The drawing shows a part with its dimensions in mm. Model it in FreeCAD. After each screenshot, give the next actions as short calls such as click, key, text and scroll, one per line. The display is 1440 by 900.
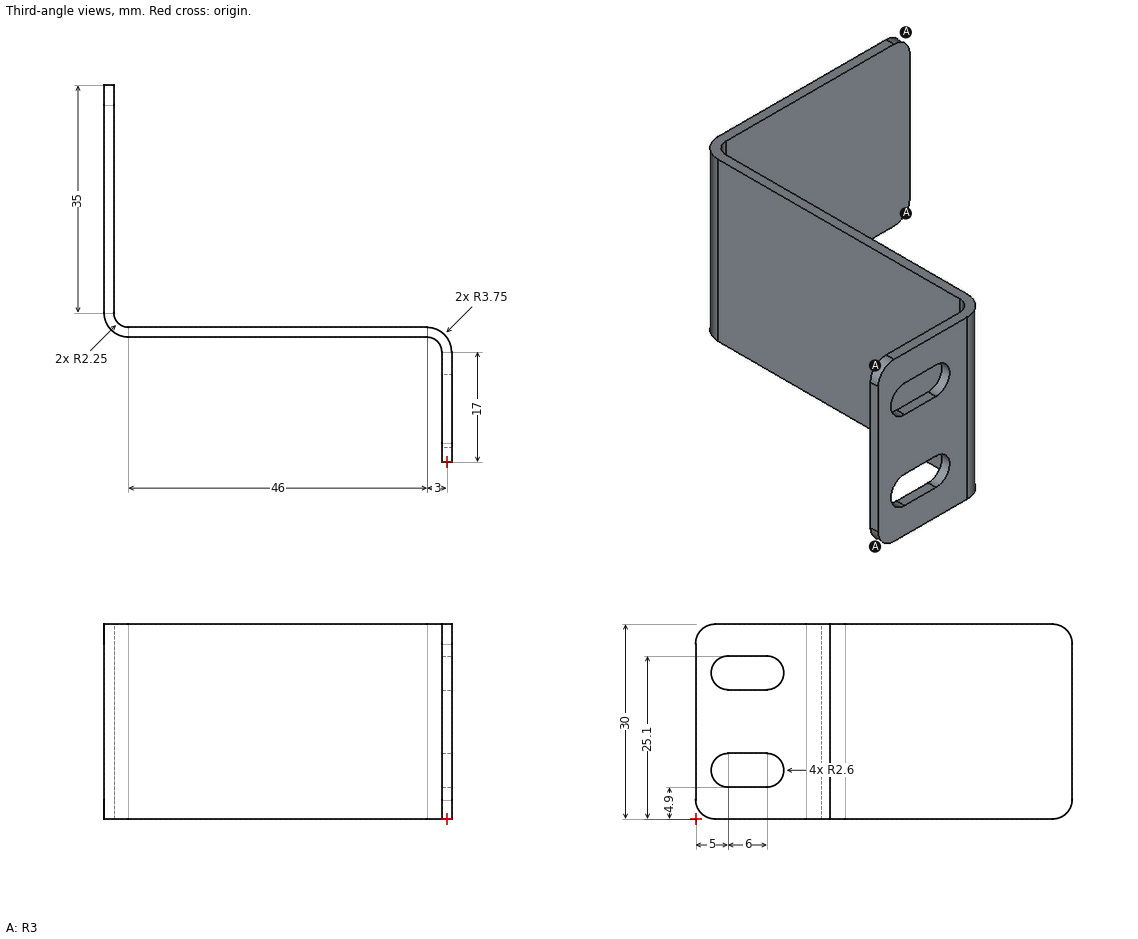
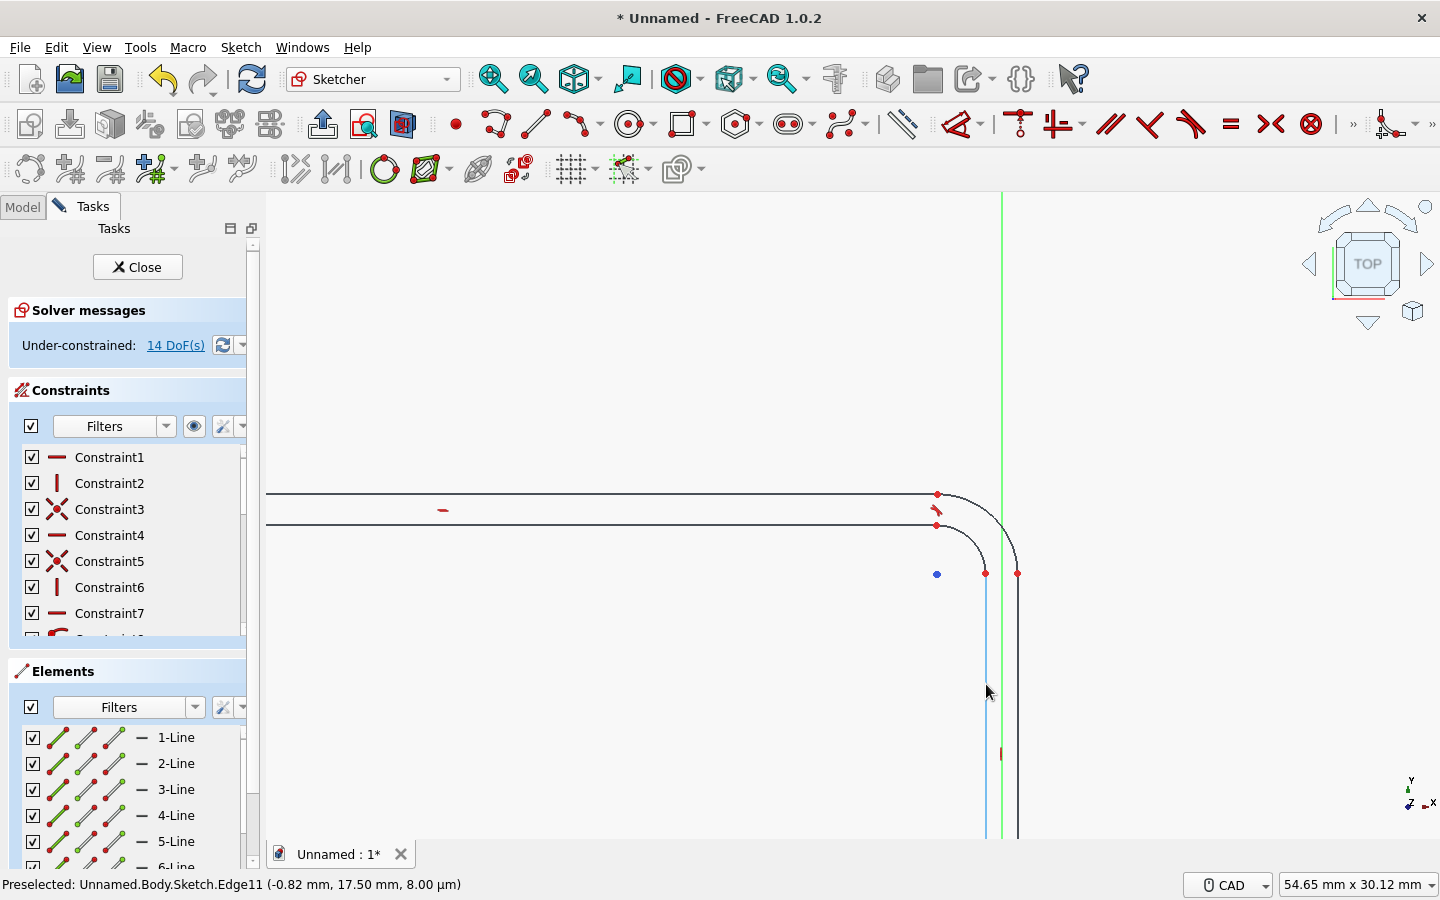
click(986, 683)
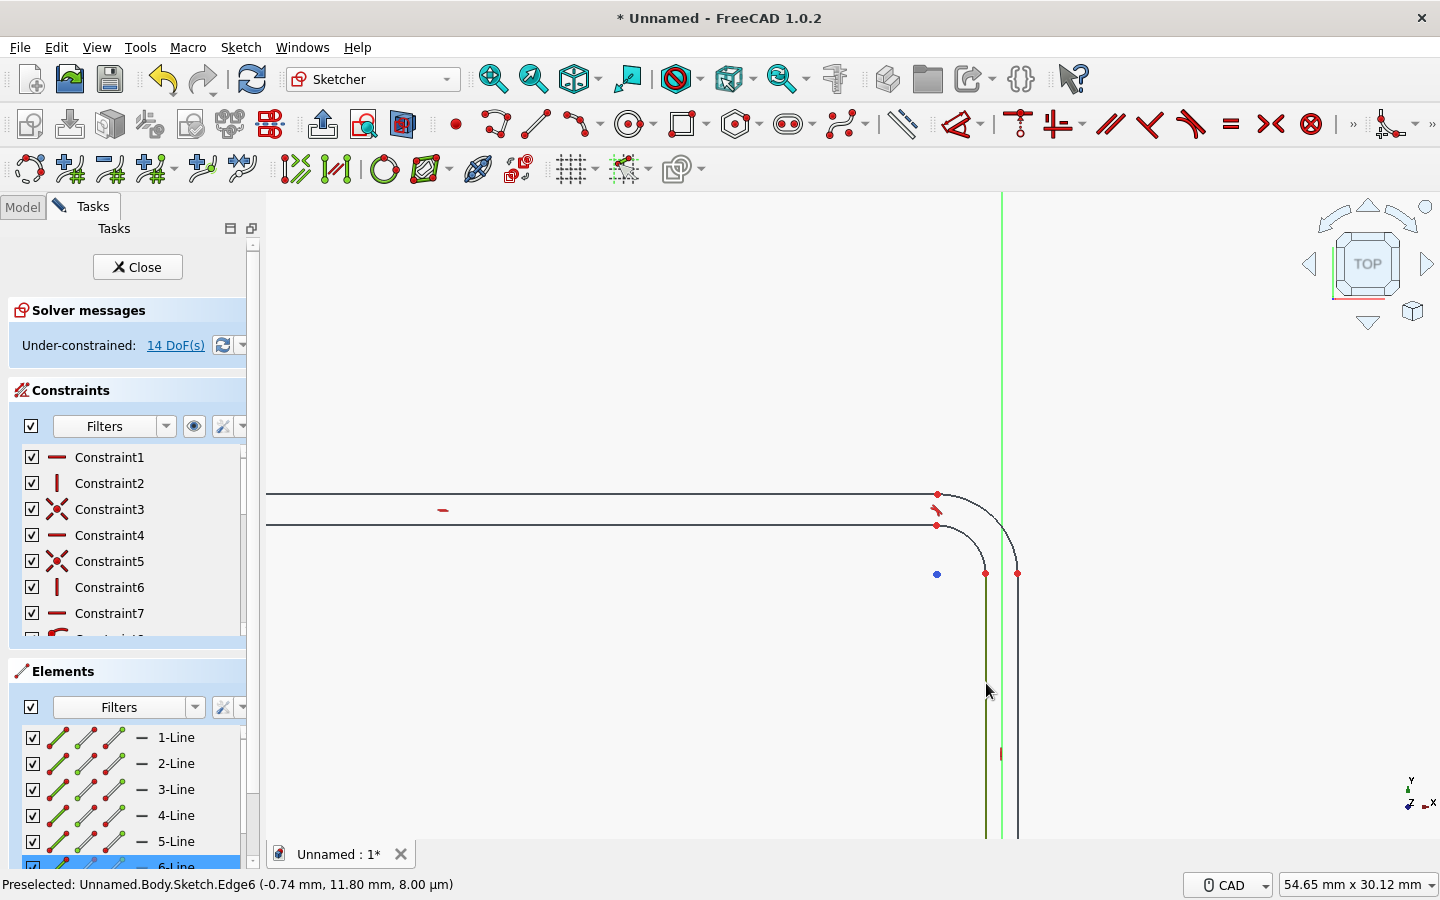
click(980, 552)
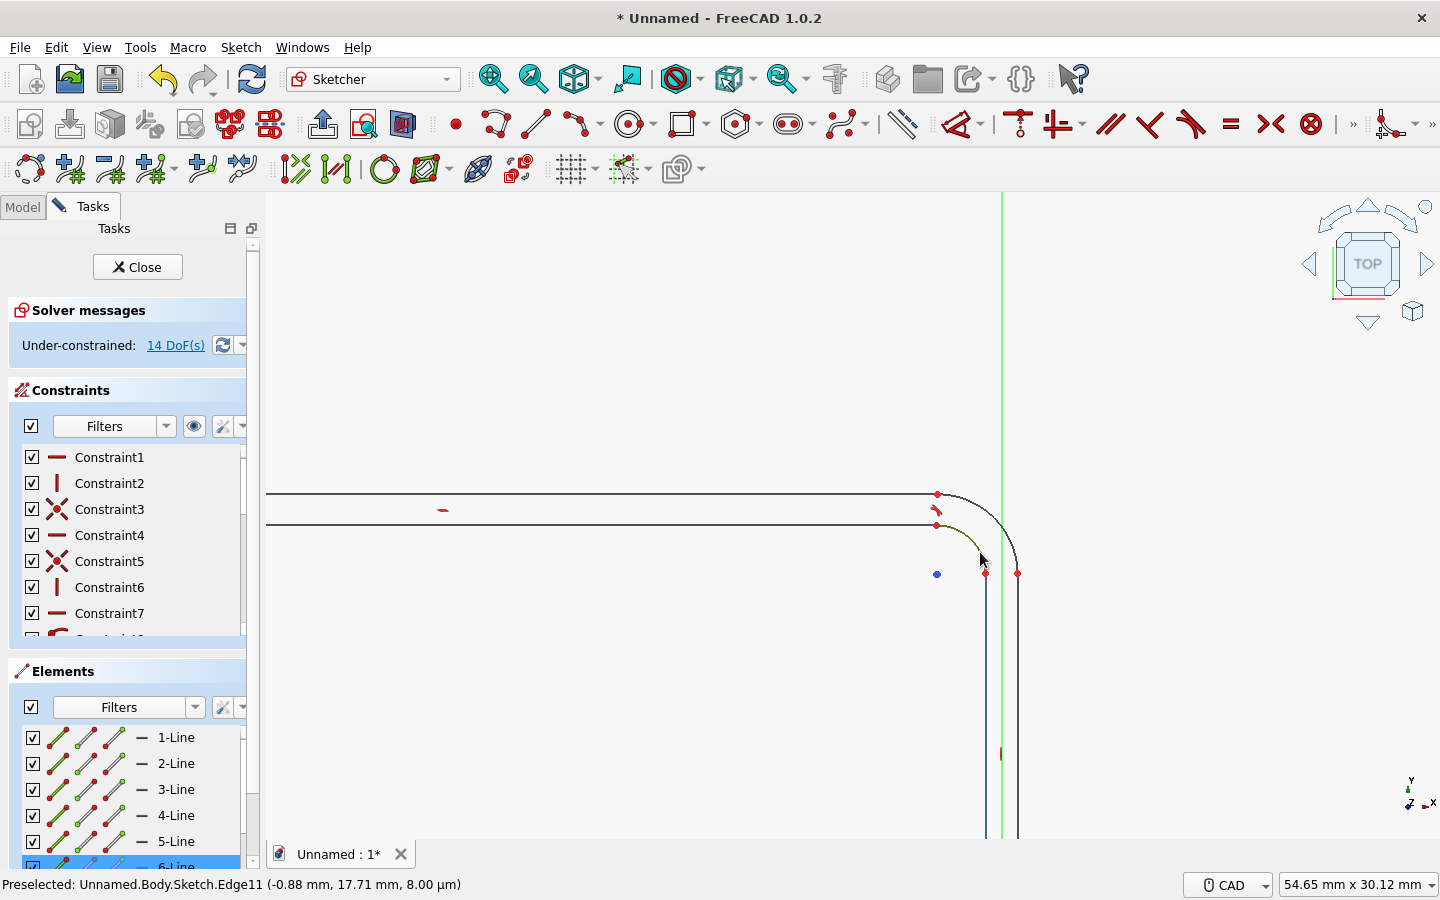
key(t)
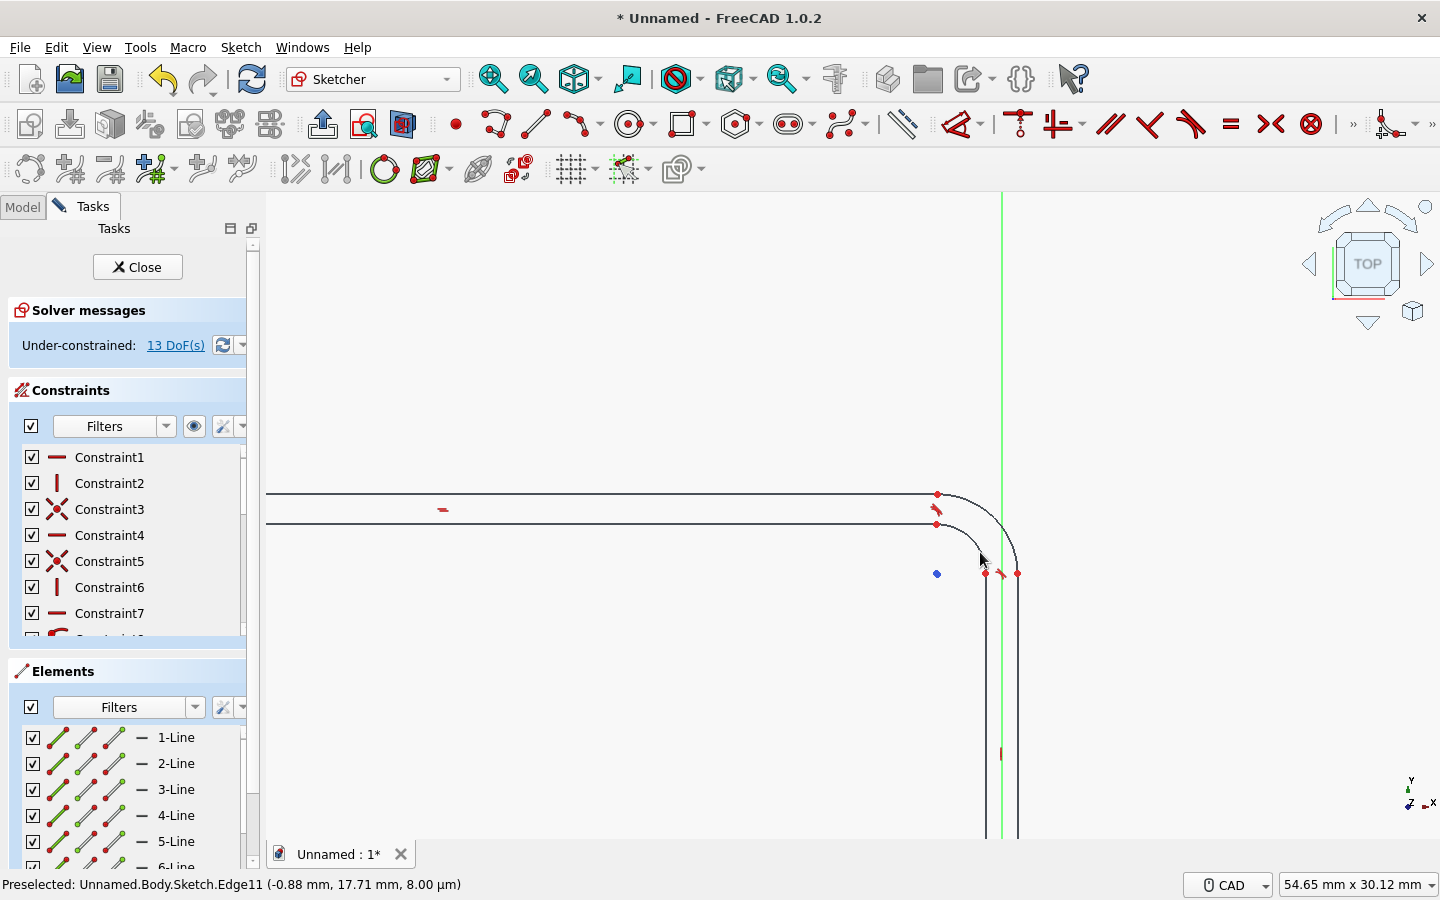
click(1018, 681)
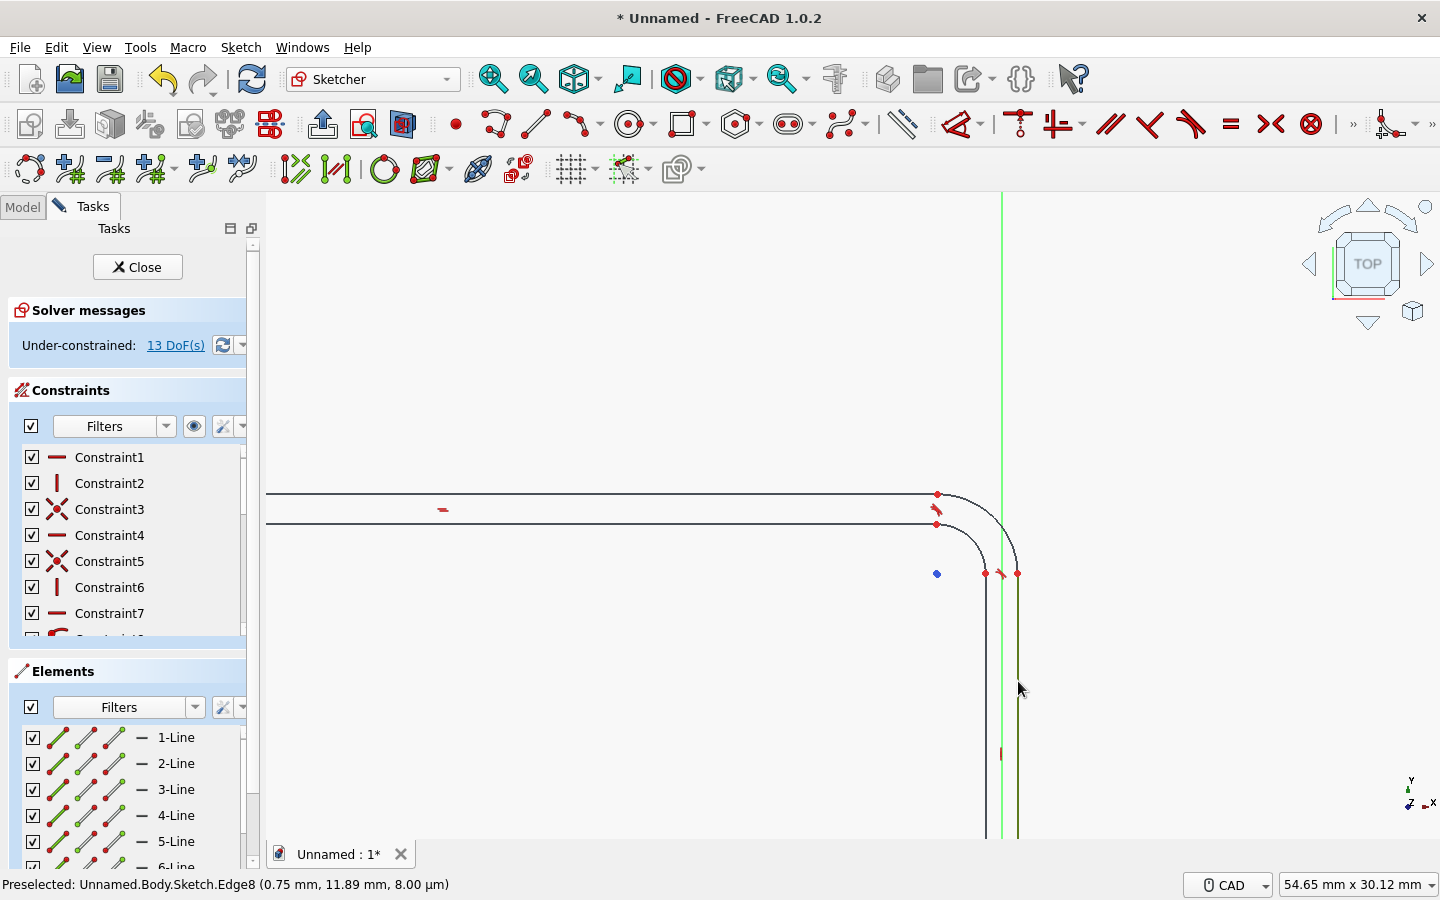
click(973, 503)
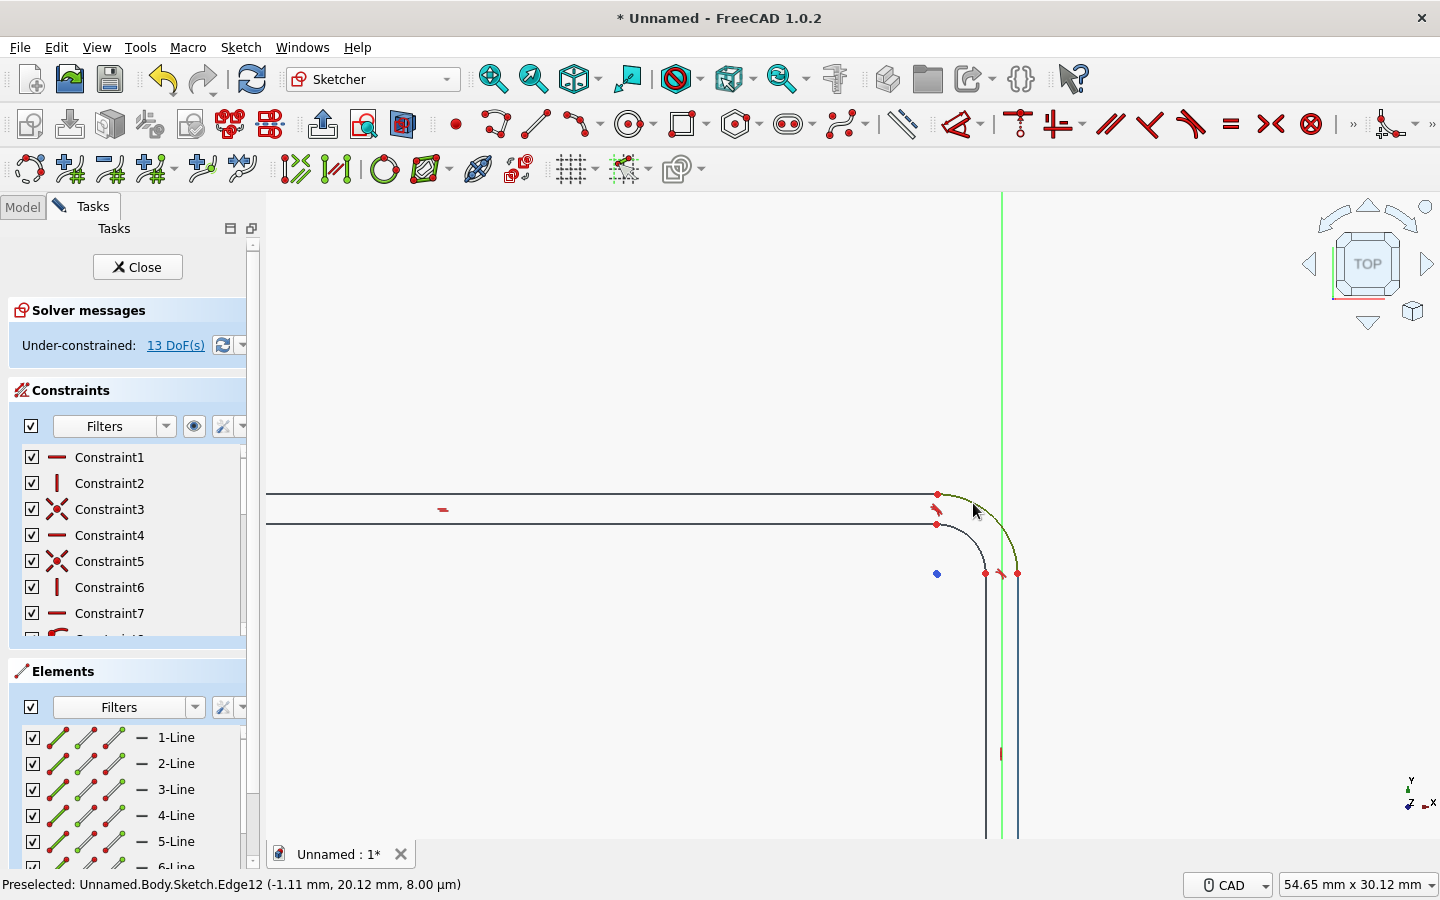
click(1192, 124)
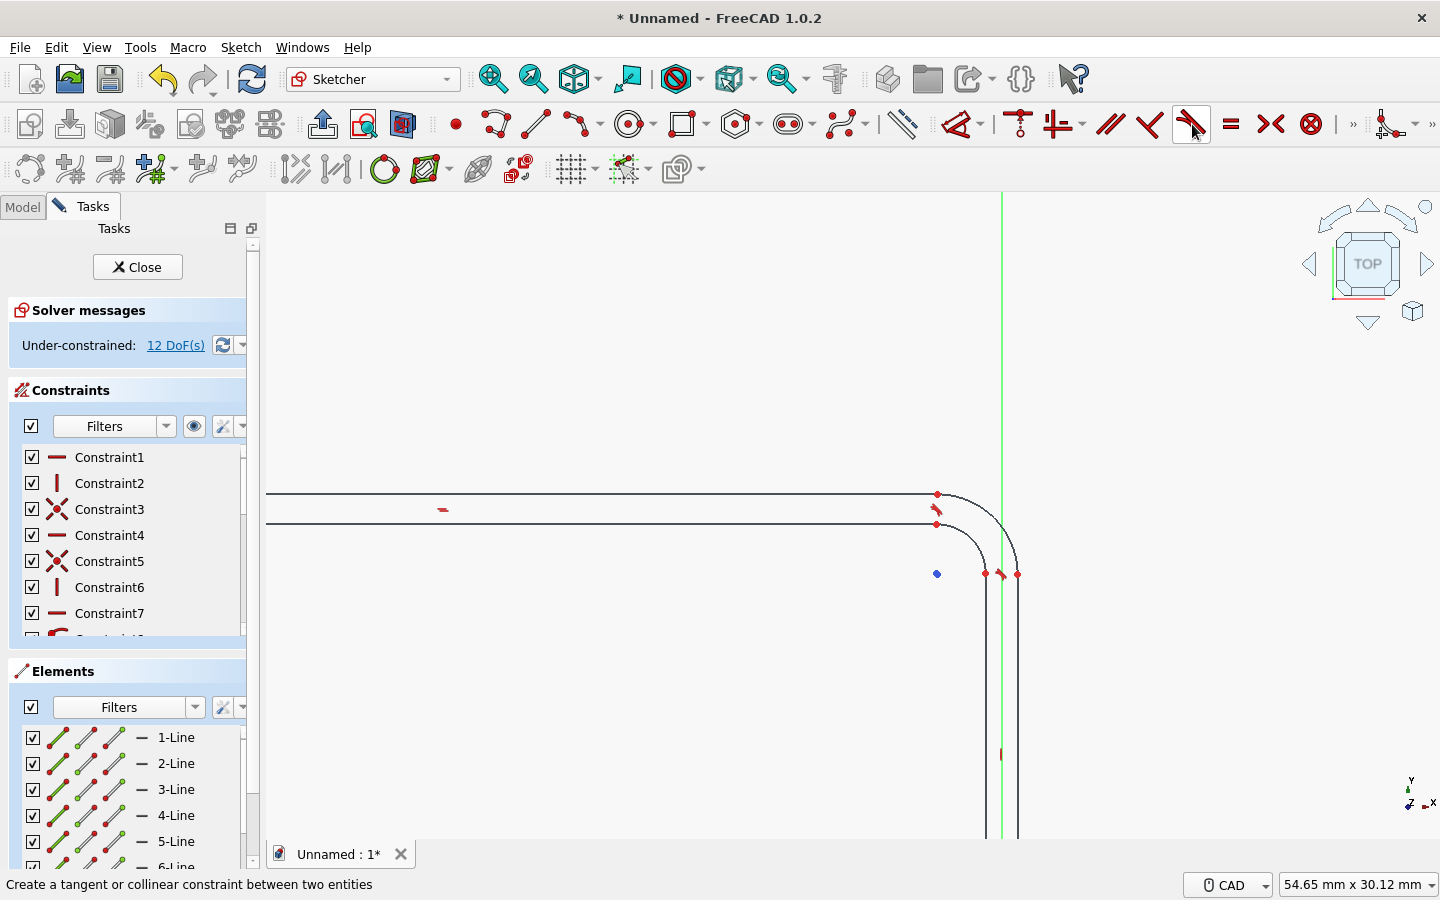
scroll(983, 632, down, 5)